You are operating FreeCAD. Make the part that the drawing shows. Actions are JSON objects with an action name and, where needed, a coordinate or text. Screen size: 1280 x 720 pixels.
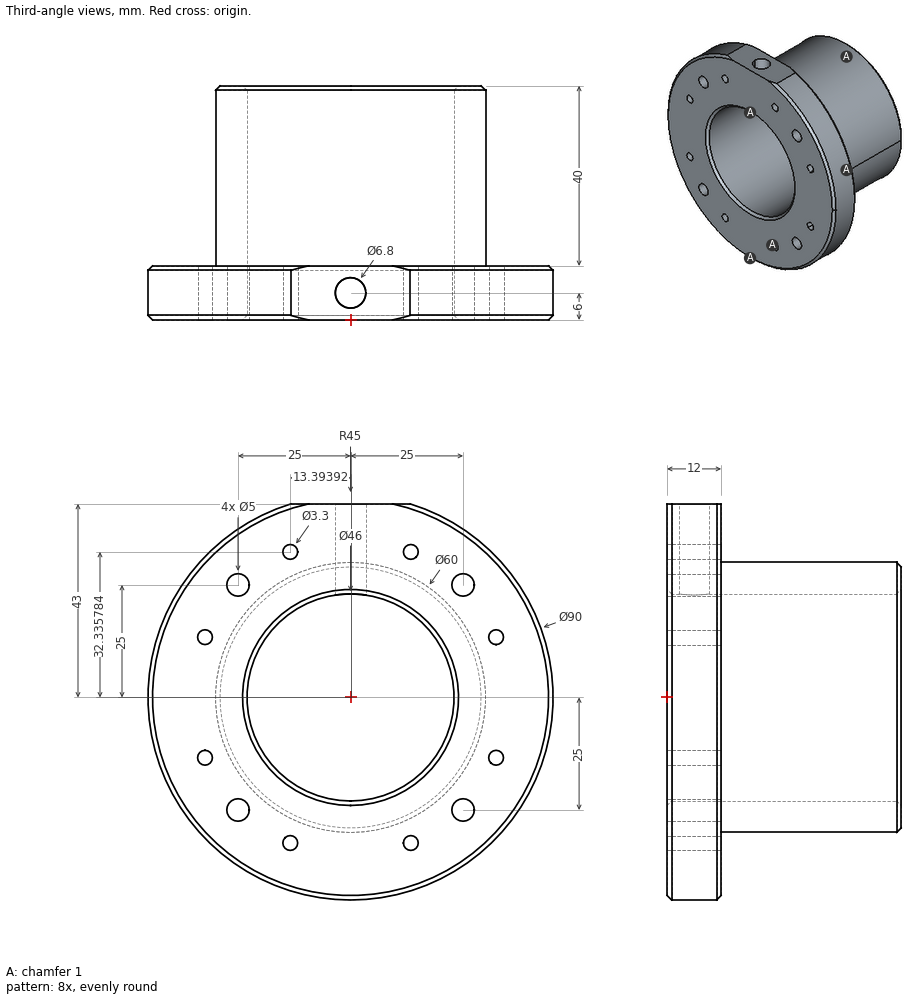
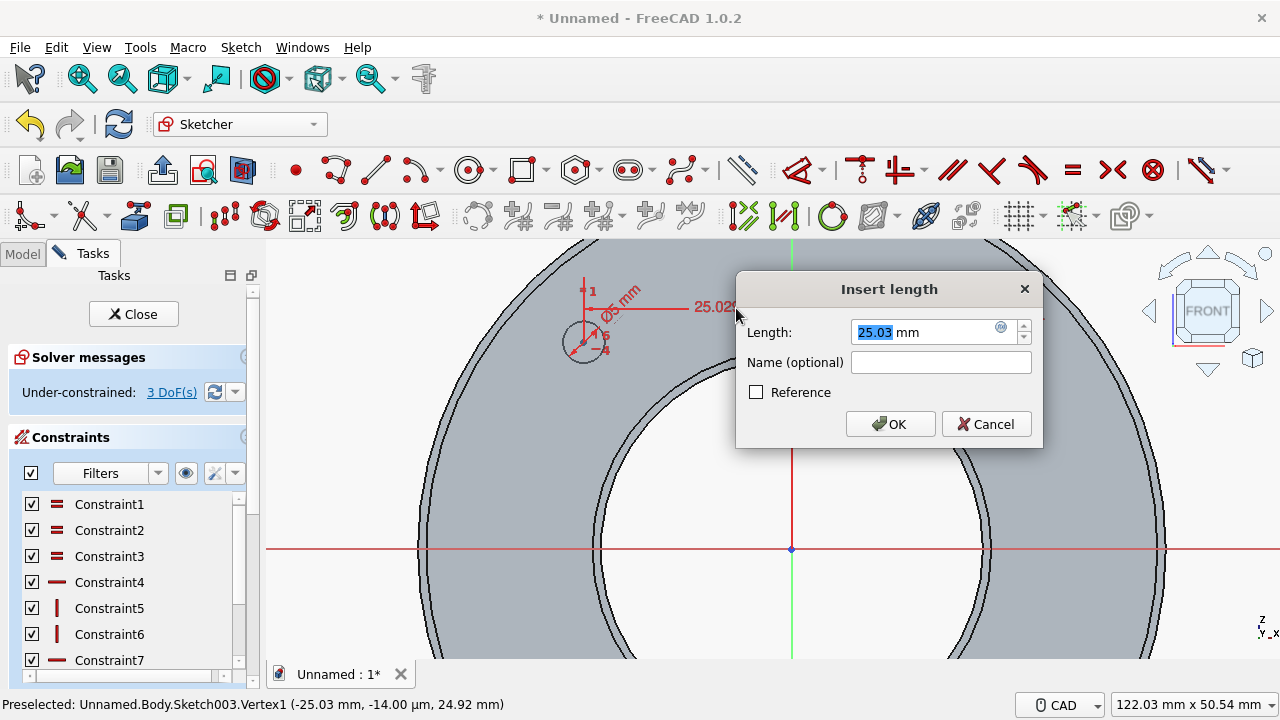
{"action": "type", "text": "25"}
{"action": "key", "text": "Return"}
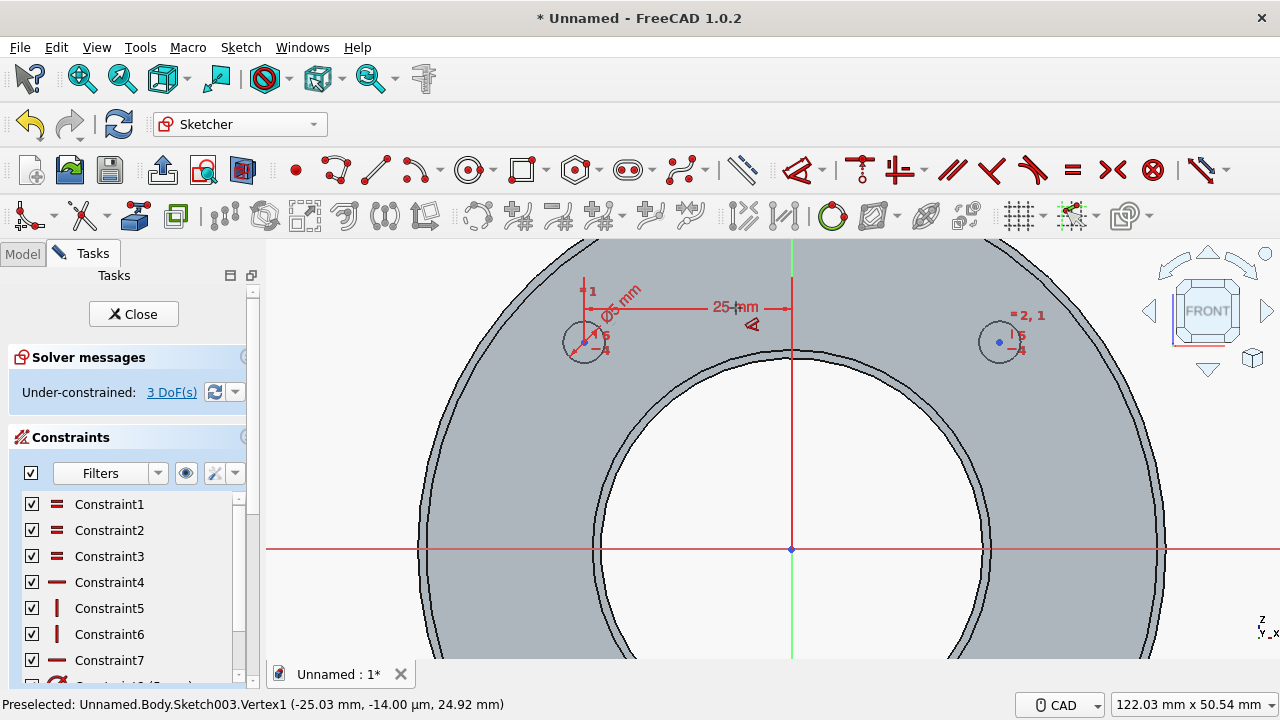
{"action": "left_click", "coordinate": [584, 342]}
{"action": "left_click", "coordinate": [550, 446]}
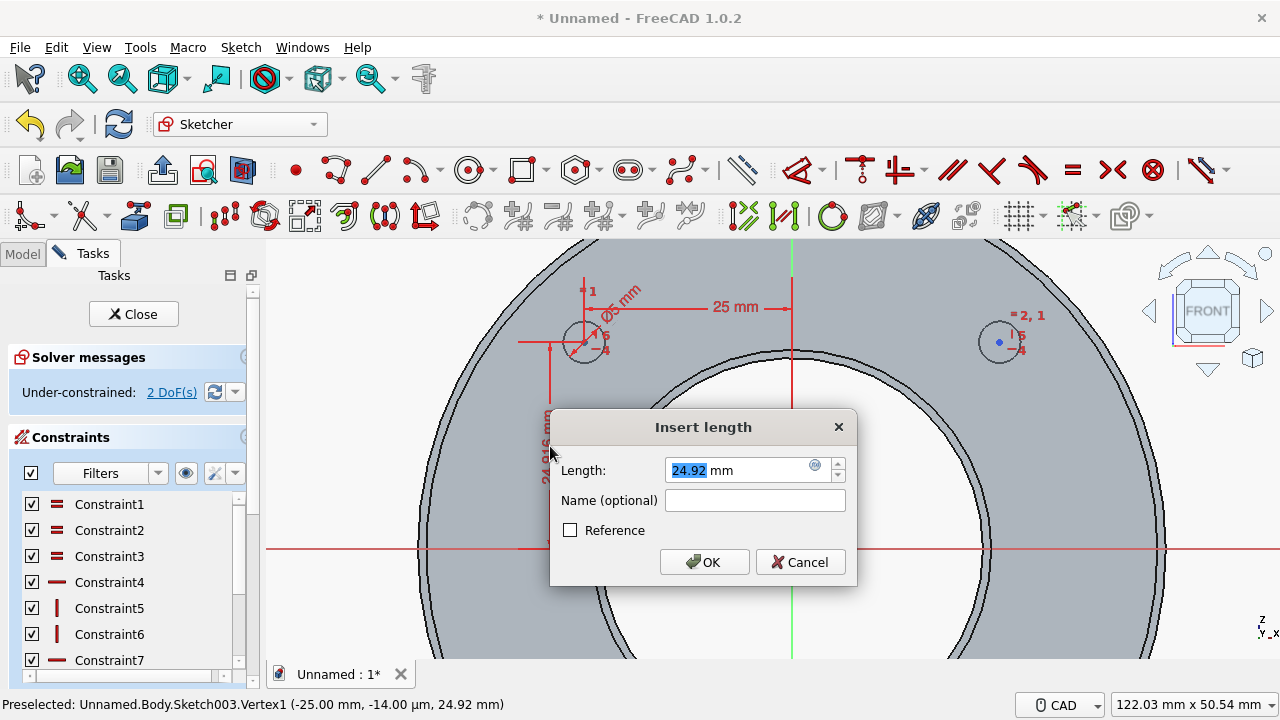
{"action": "type", "text": "25"}
{"action": "key", "text": "Return"}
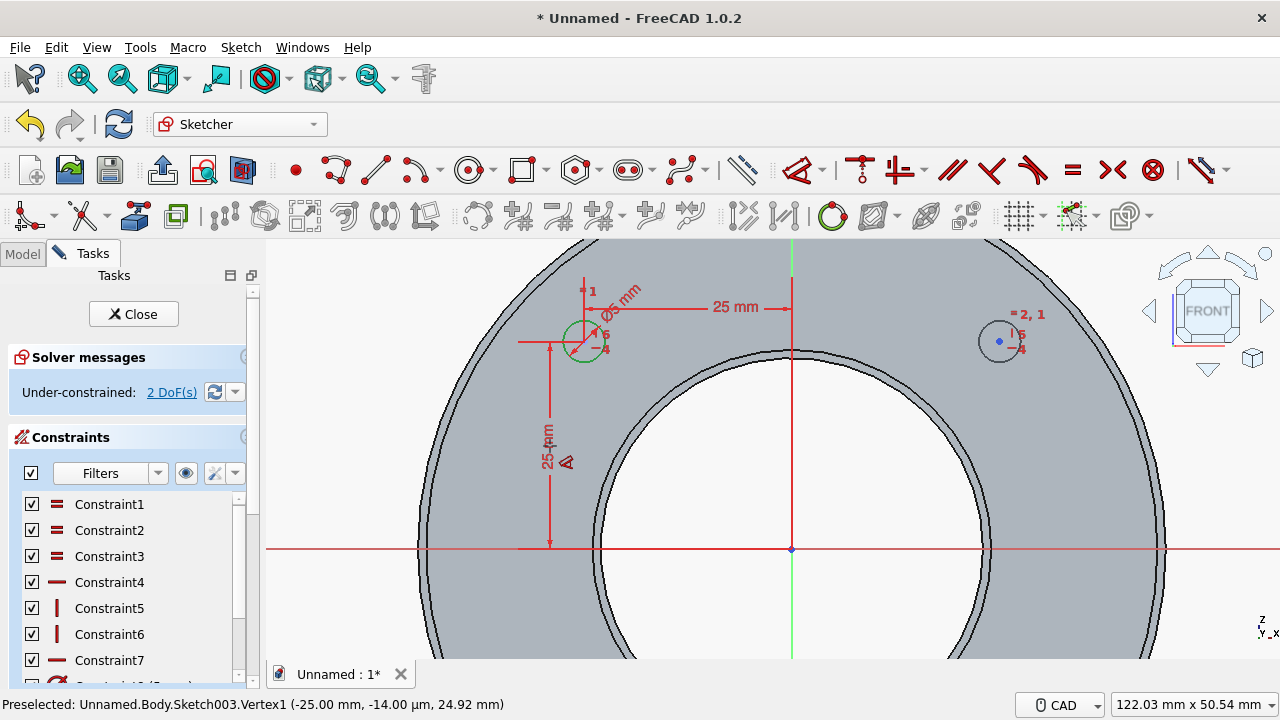
{"action": "left_click", "coordinate": [1000, 342]}
{"action": "left_click", "coordinate": [896, 308]}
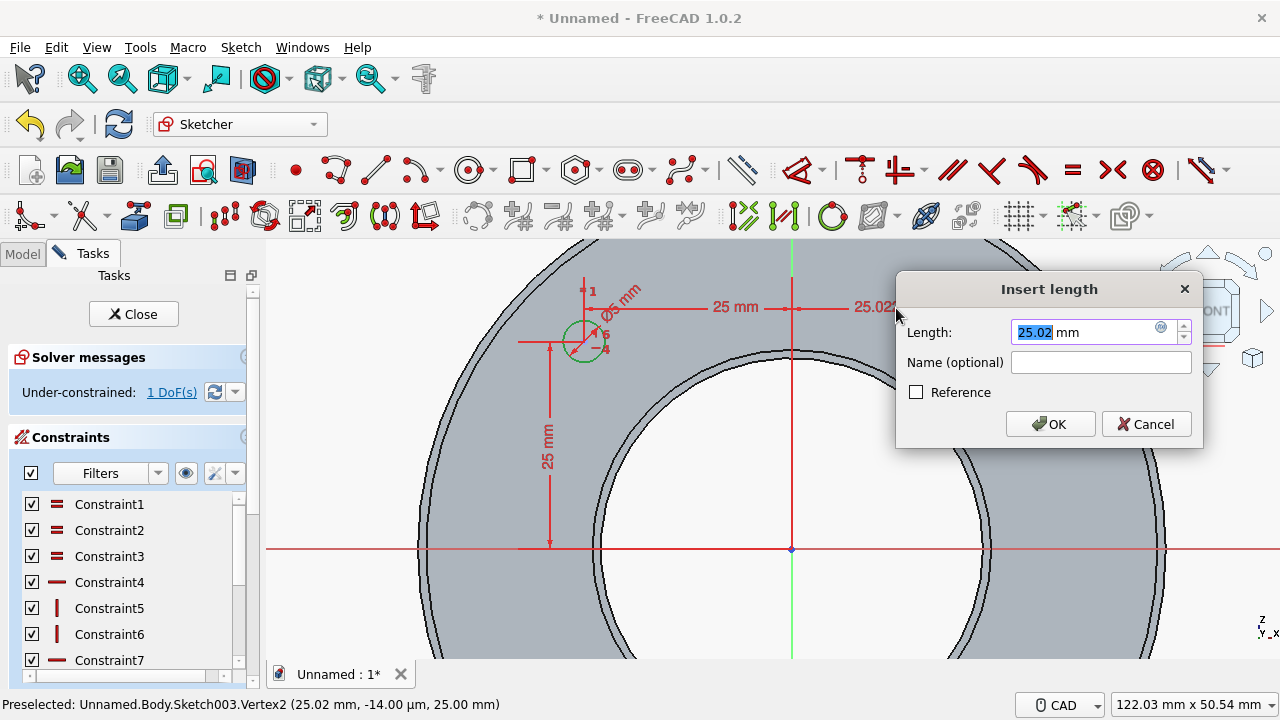
{"action": "type", "text": "25"}
{"action": "key", "text": "Return"}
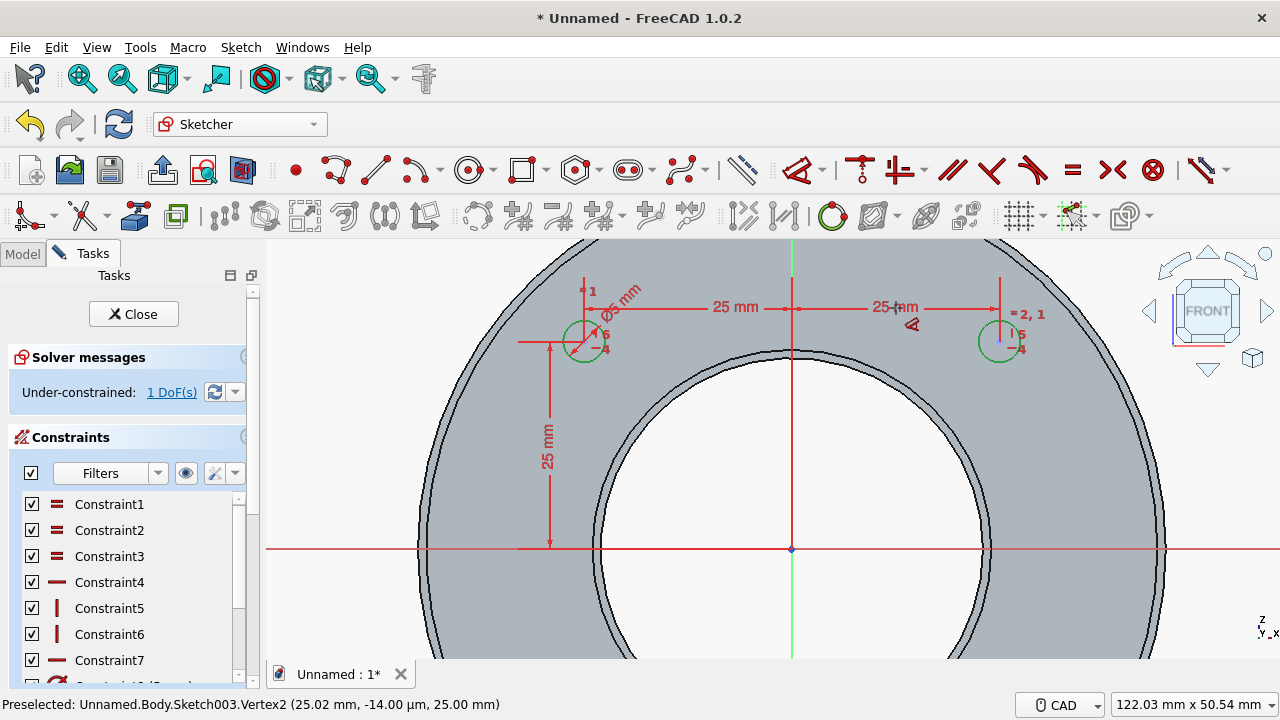
{"action": "scroll", "coordinate": [598, 327], "scroll_direction": "down", "scroll_amount": 3}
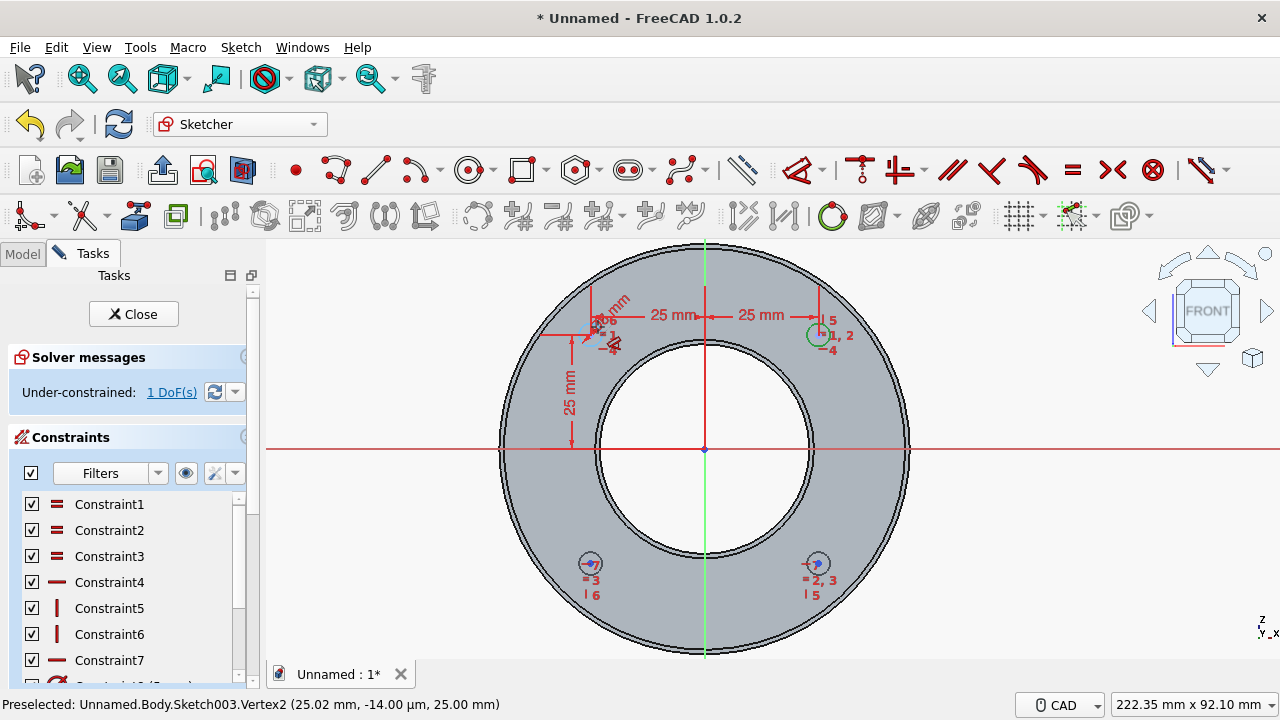
{"action": "left_click", "coordinate": [819, 564]}
{"action": "left_click", "coordinate": [853, 506]}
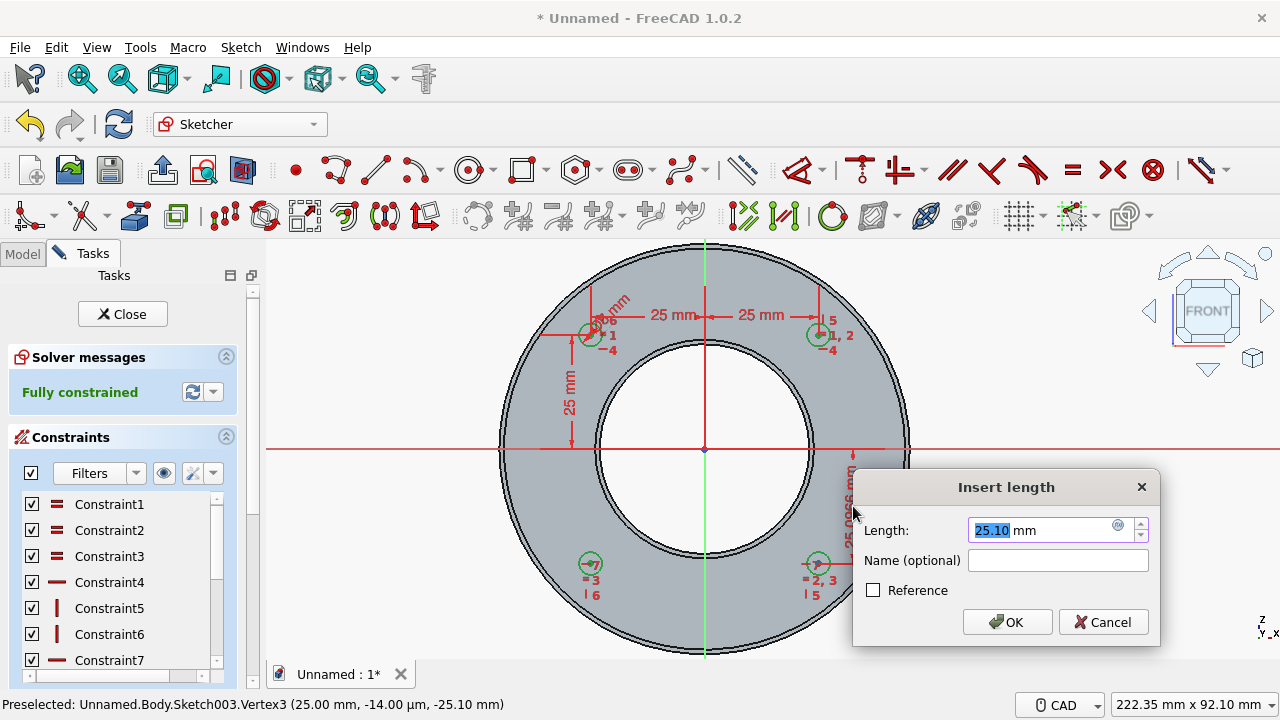
{"action": "type", "text": "25"}
{"action": "key", "text": "Return"}
{"action": "key", "text": "Escape"}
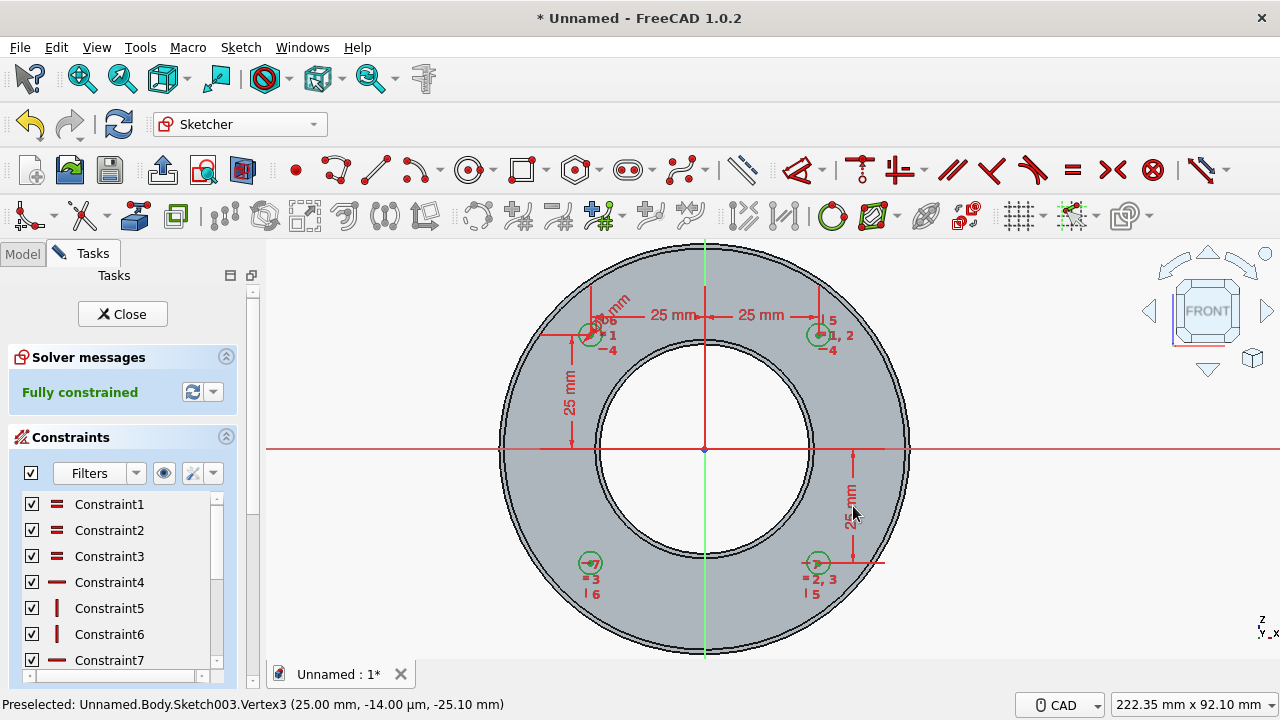
{"action": "left_click", "coordinate": [123, 314]}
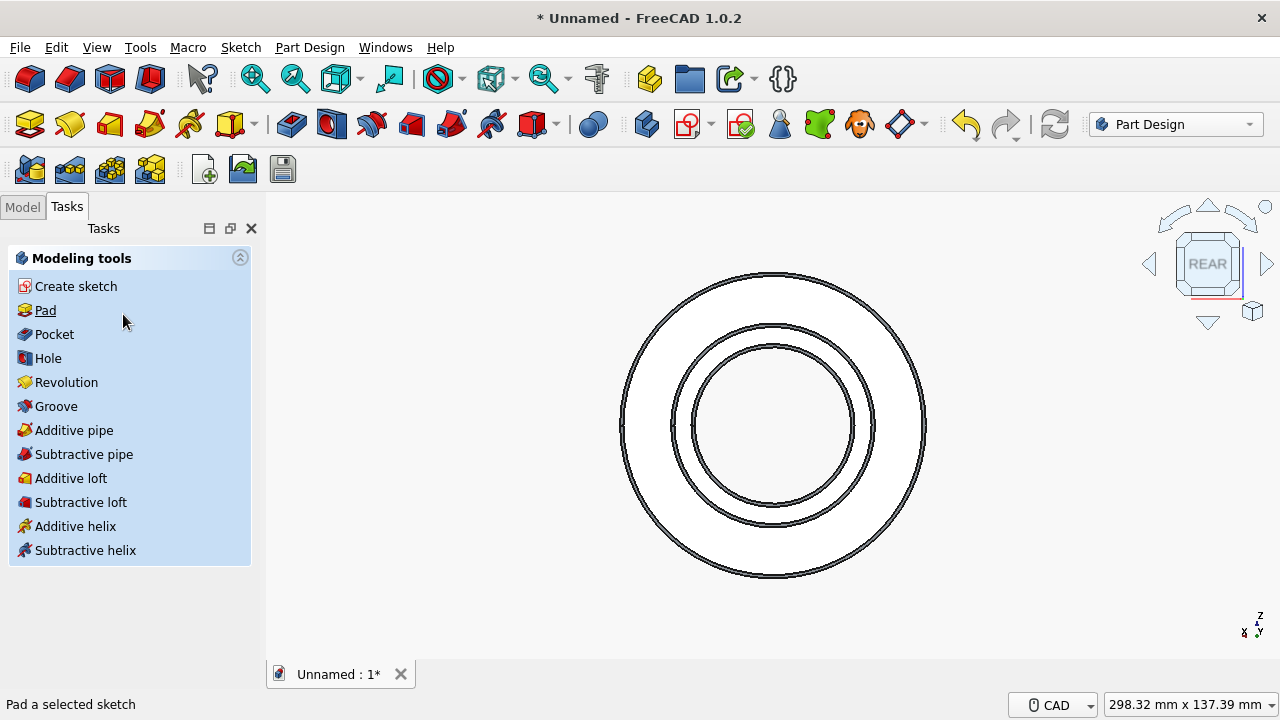
{"action": "left_click", "coordinate": [292, 124]}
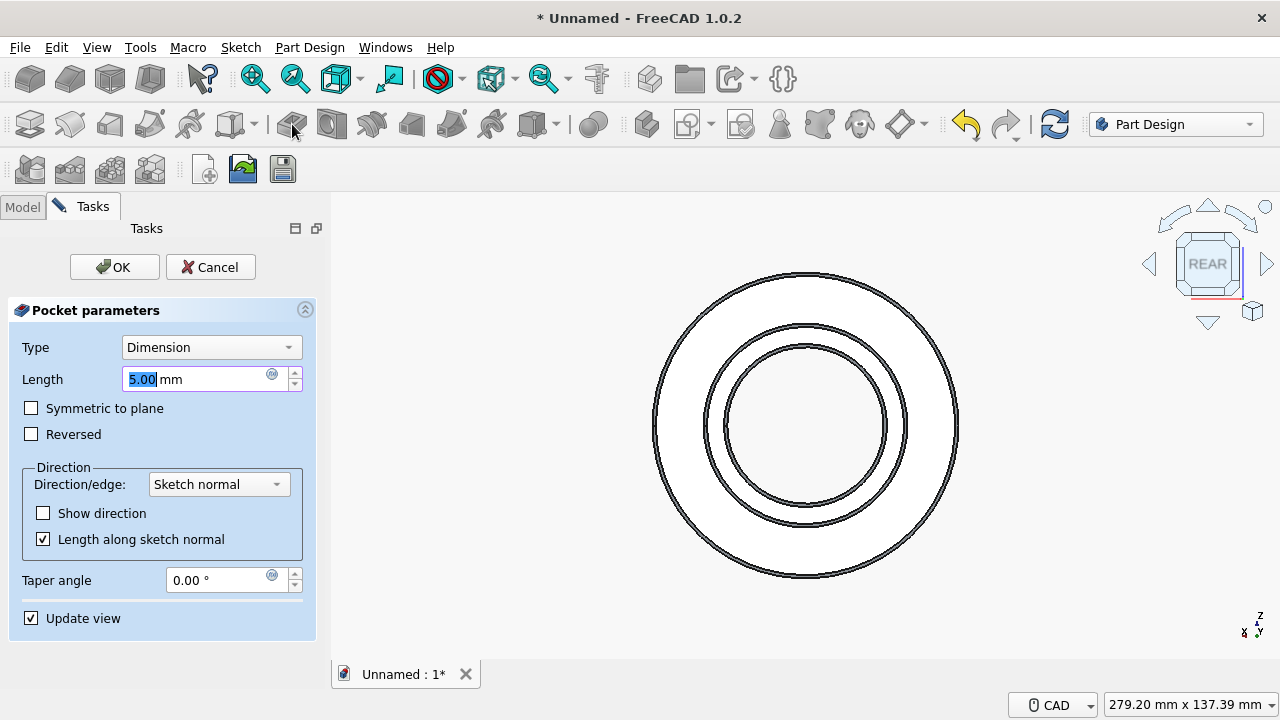
{"action": "left_click", "coordinate": [212, 348]}